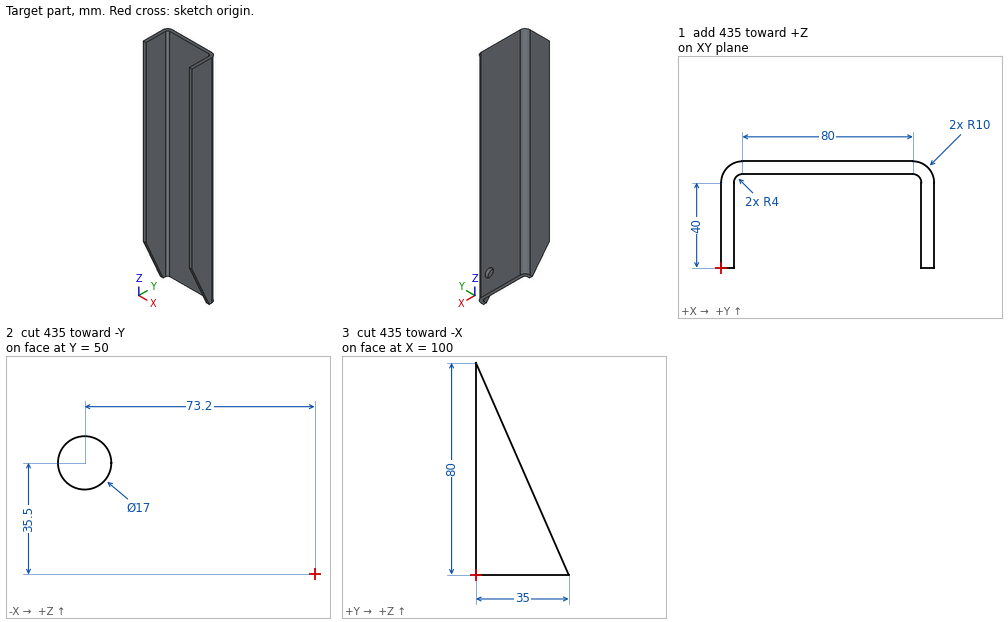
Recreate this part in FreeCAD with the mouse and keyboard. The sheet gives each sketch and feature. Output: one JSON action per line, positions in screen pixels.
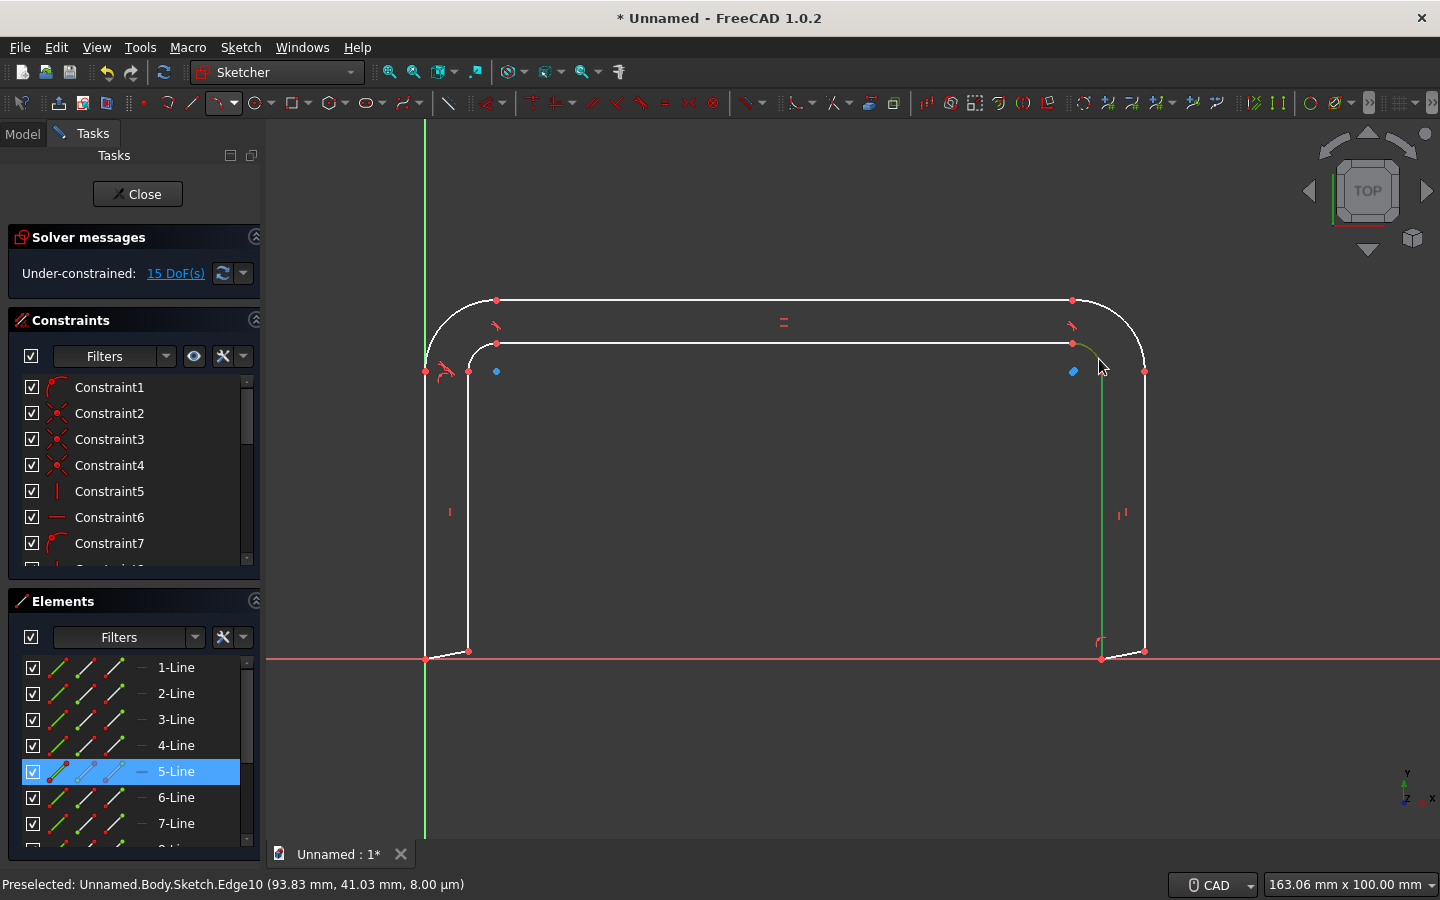
{"action": "left_click", "coordinate": [642, 104]}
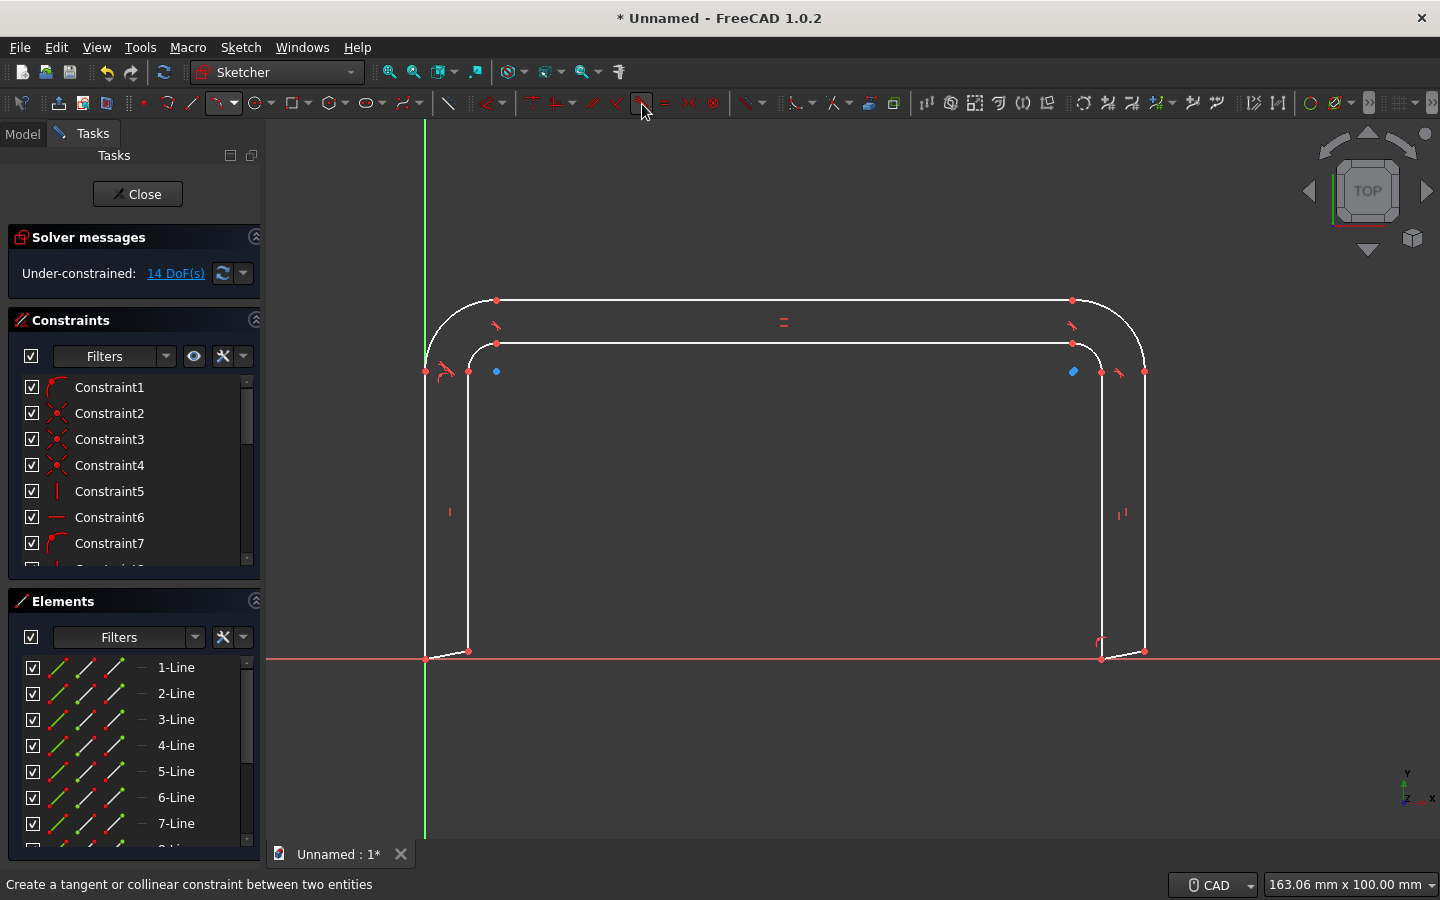
{"action": "left_click", "coordinate": [1145, 567]}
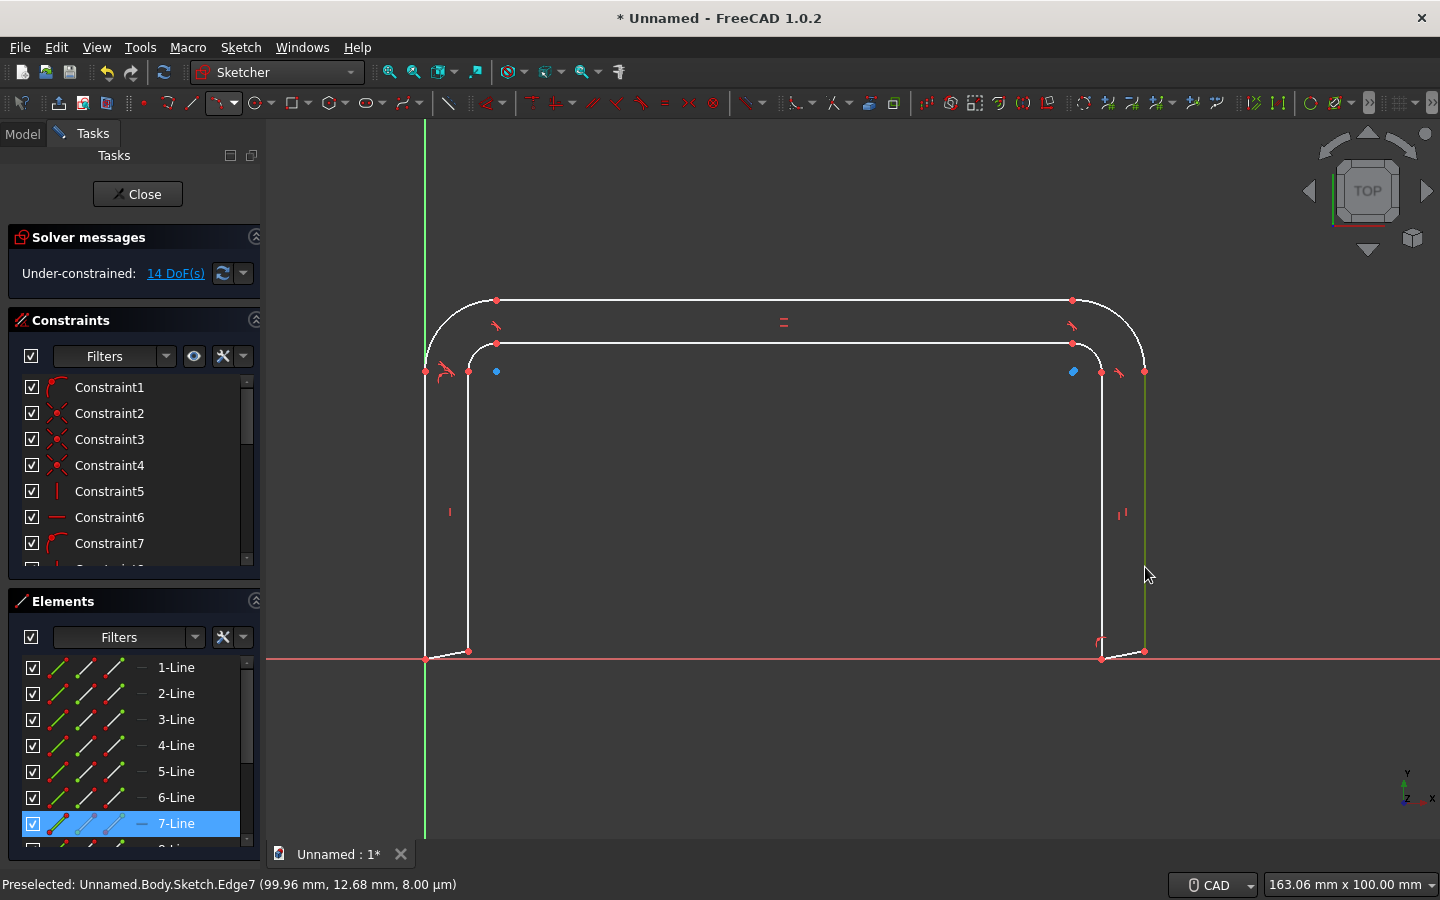
{"action": "left_click", "coordinate": [1137, 339]}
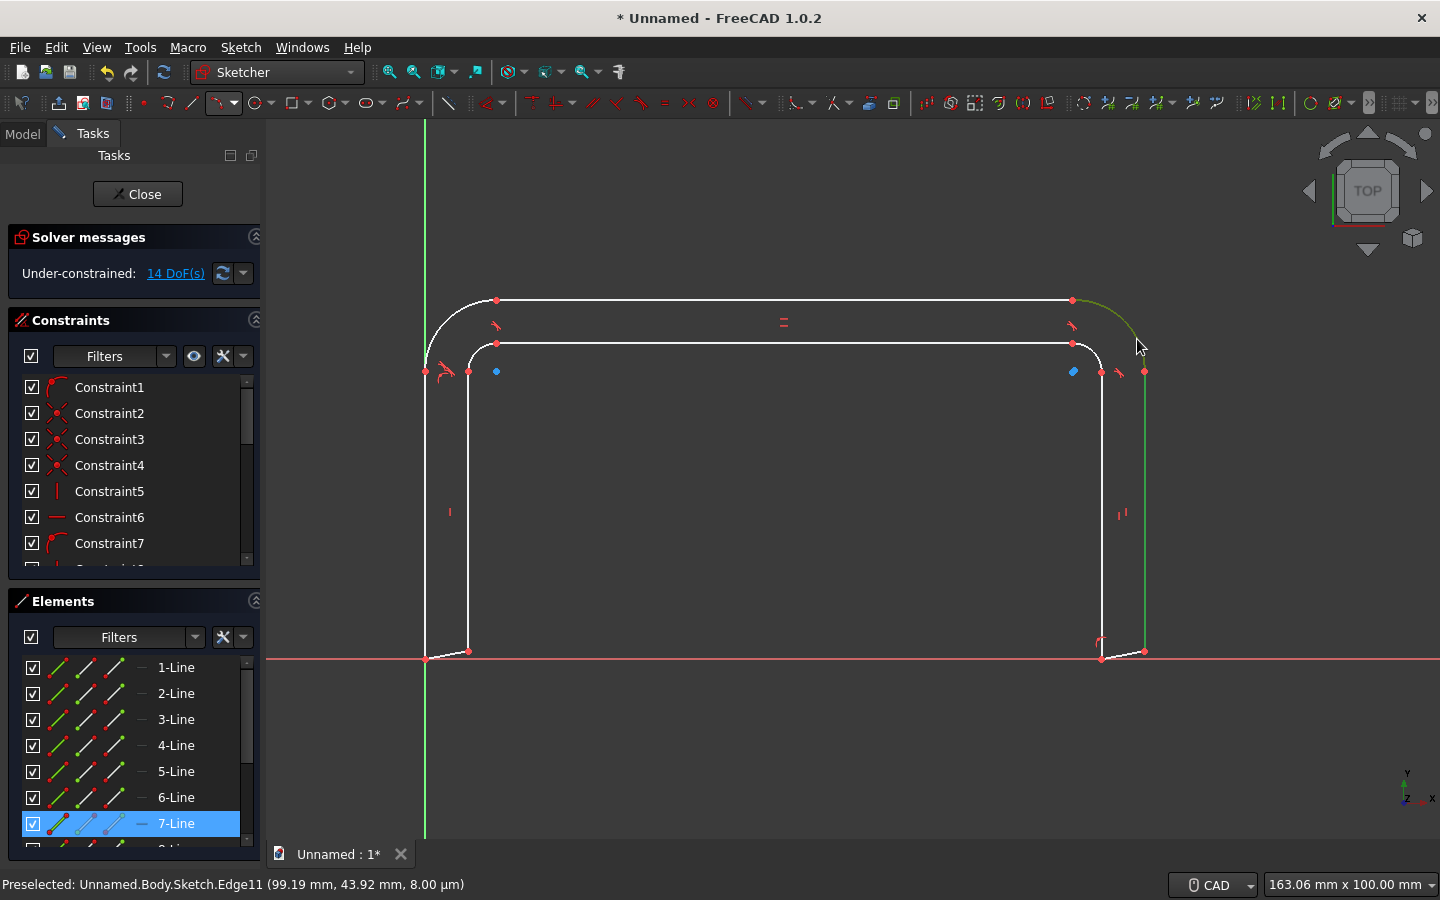
{"action": "left_click", "coordinate": [642, 104]}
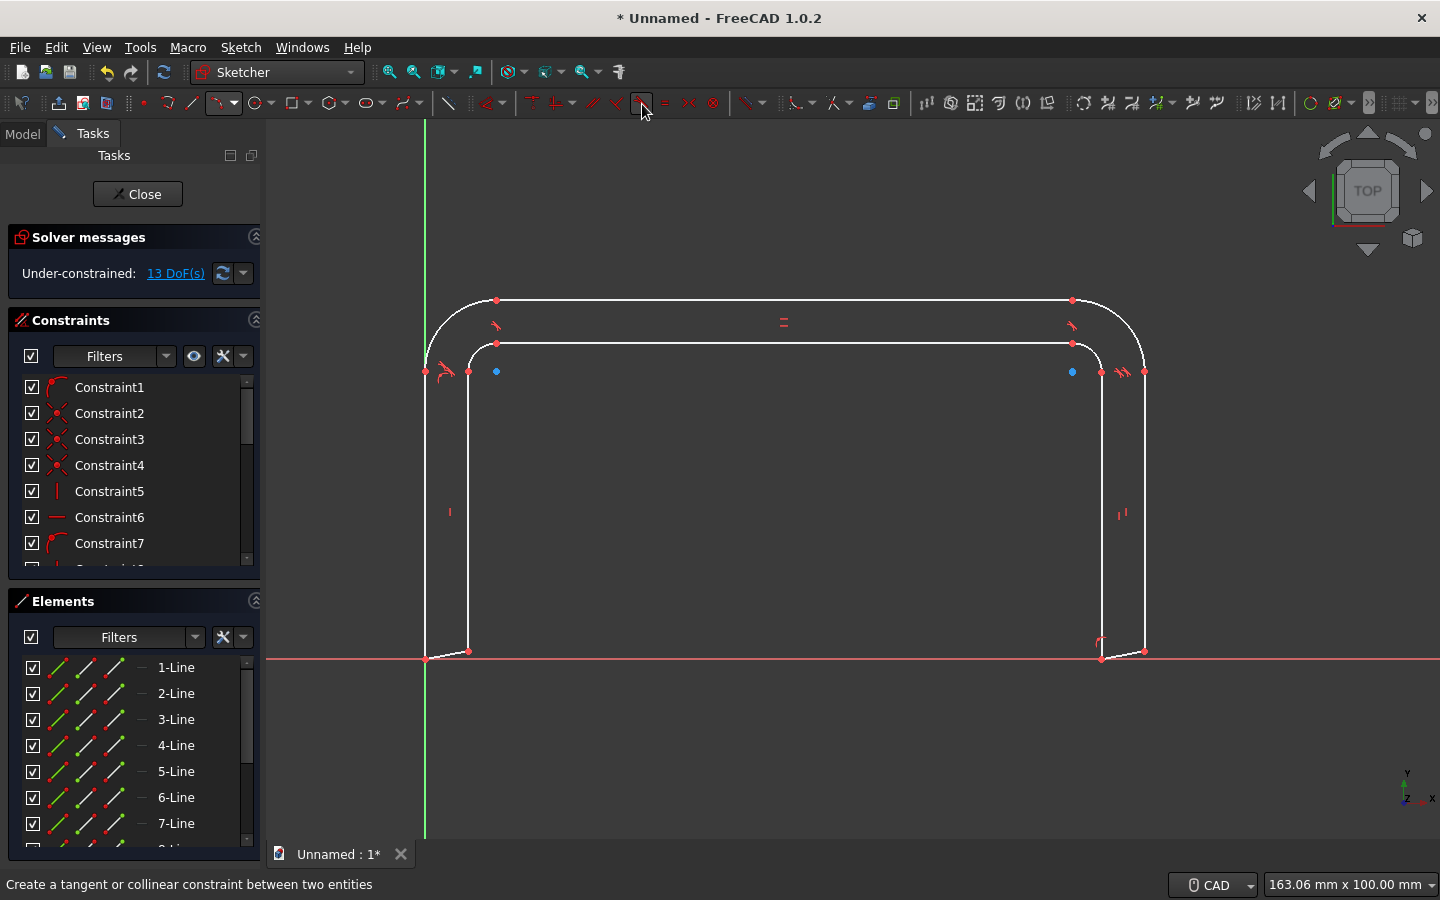
{"action": "left_click", "coordinate": [900, 300]}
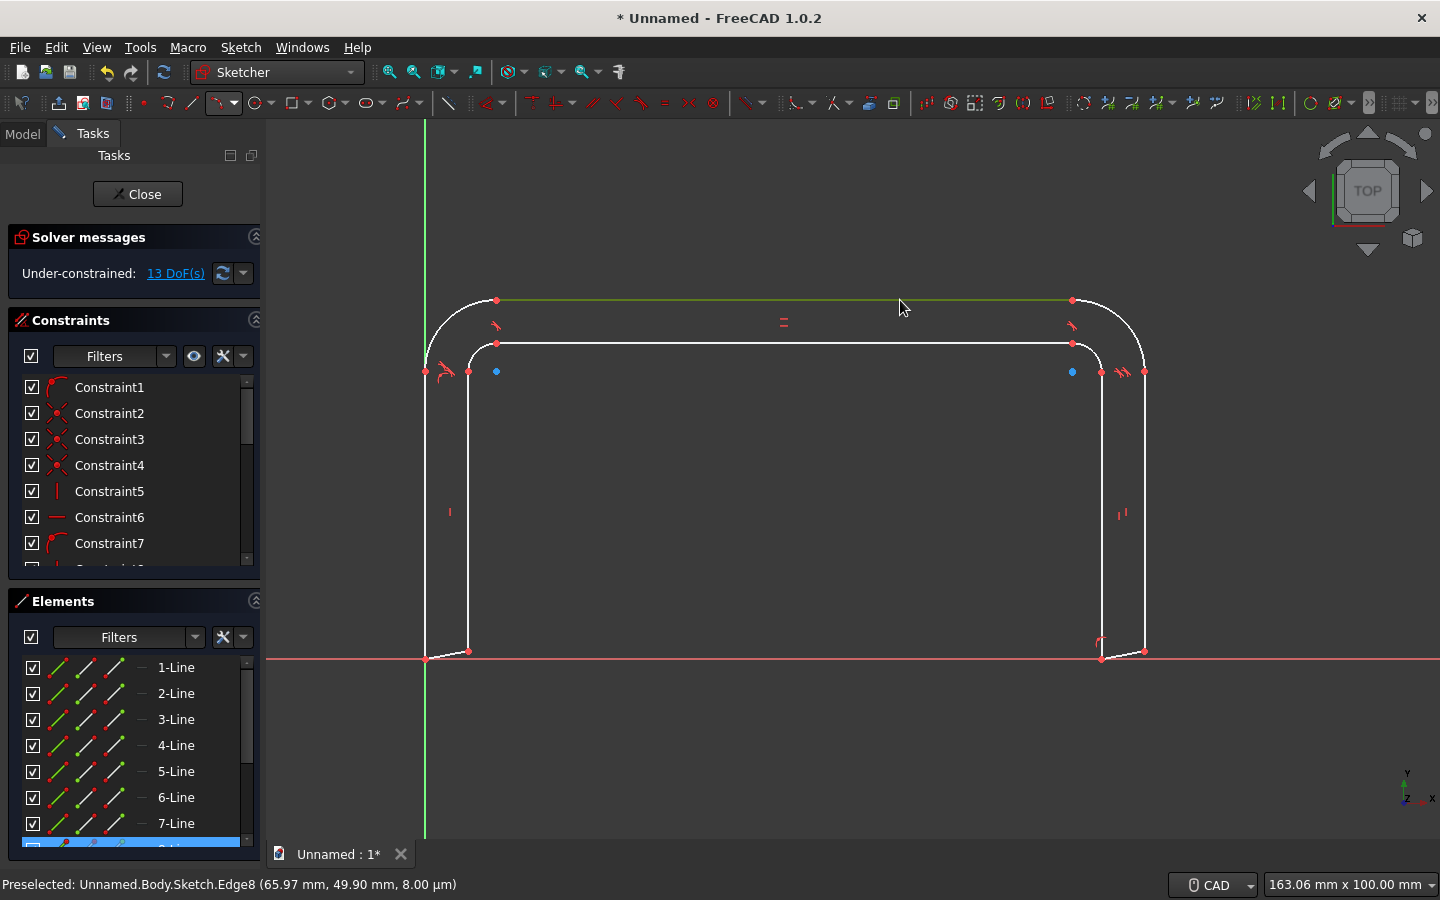
{"action": "left_click", "coordinate": [1137, 339]}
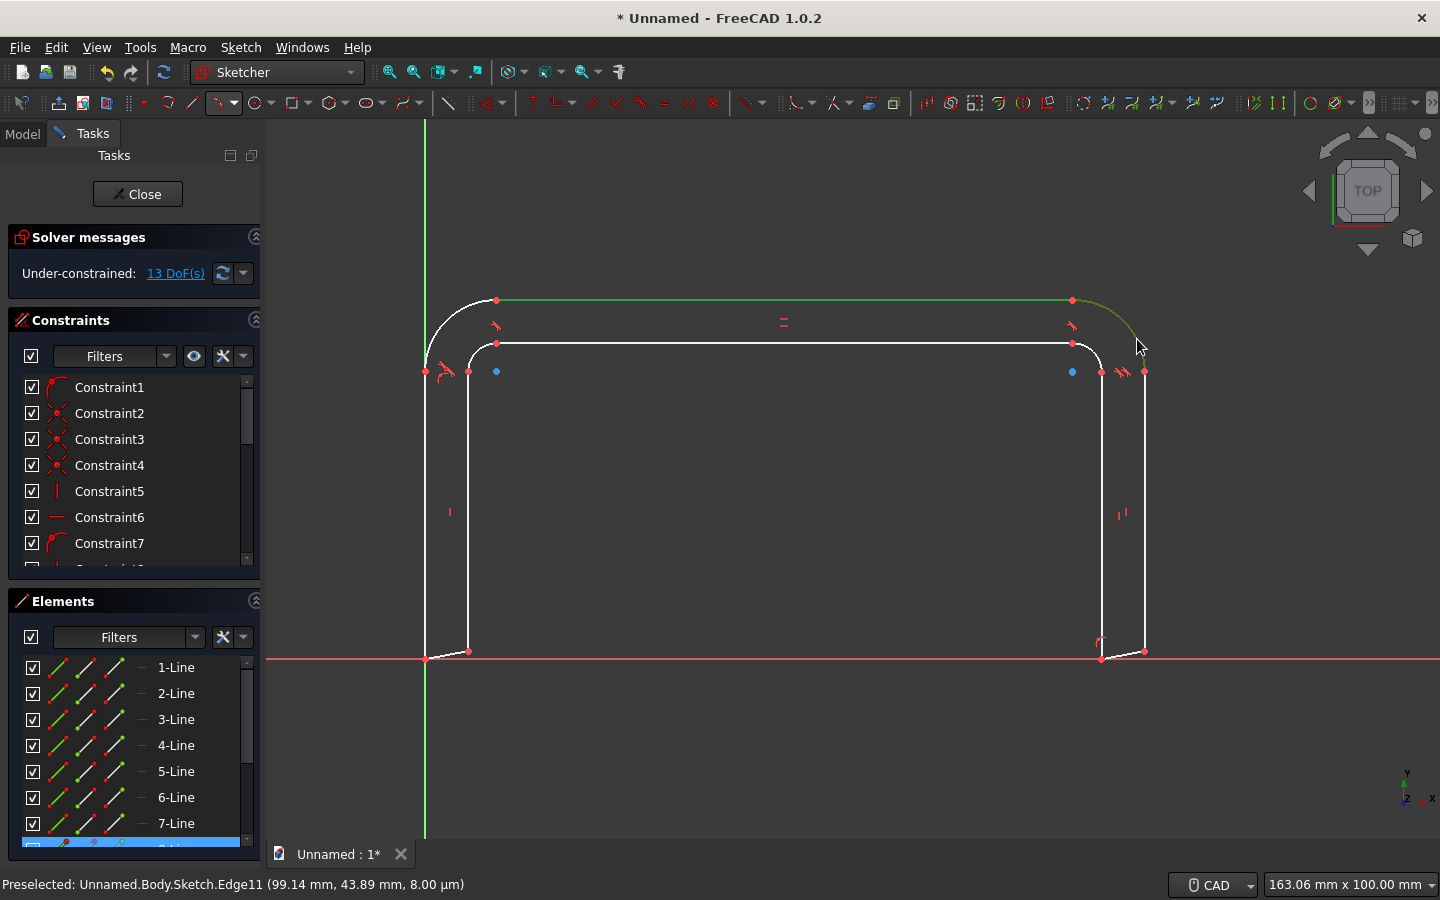
{"action": "left_click", "coordinate": [642, 104]}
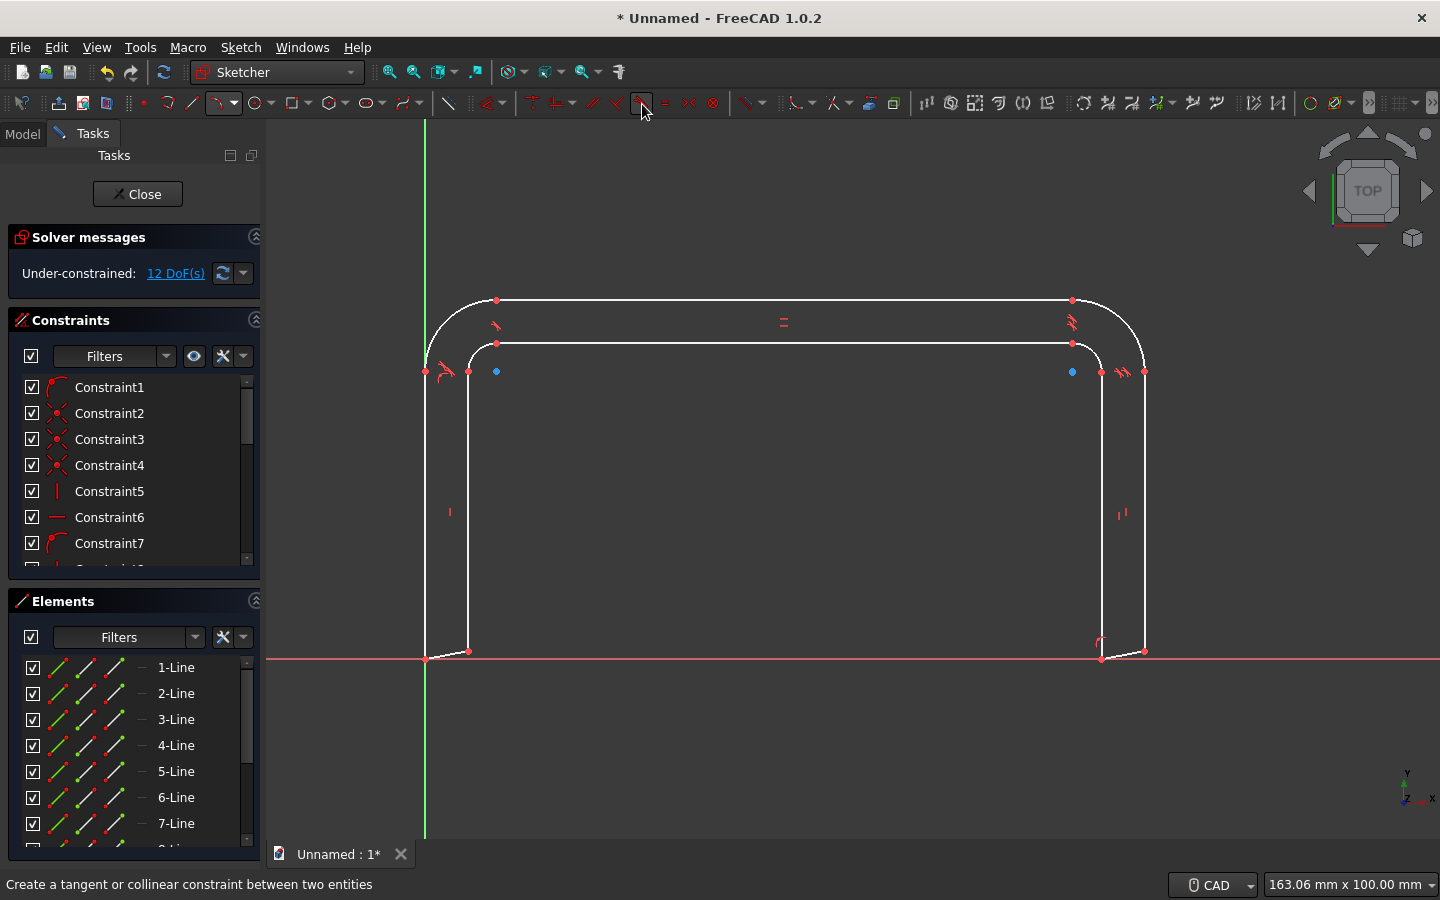
{"action": "left_click", "coordinate": [900, 300]}